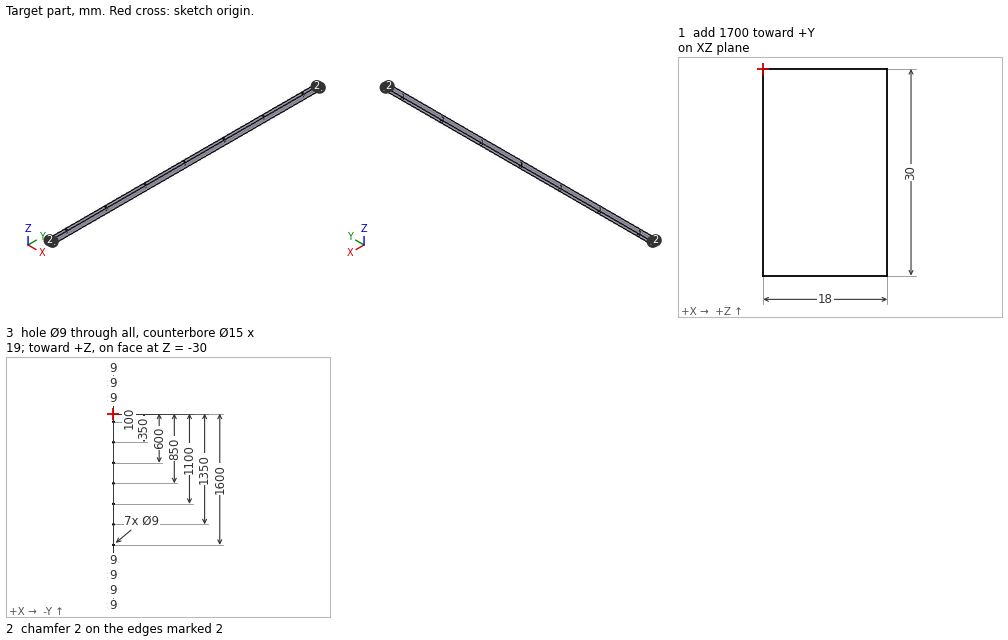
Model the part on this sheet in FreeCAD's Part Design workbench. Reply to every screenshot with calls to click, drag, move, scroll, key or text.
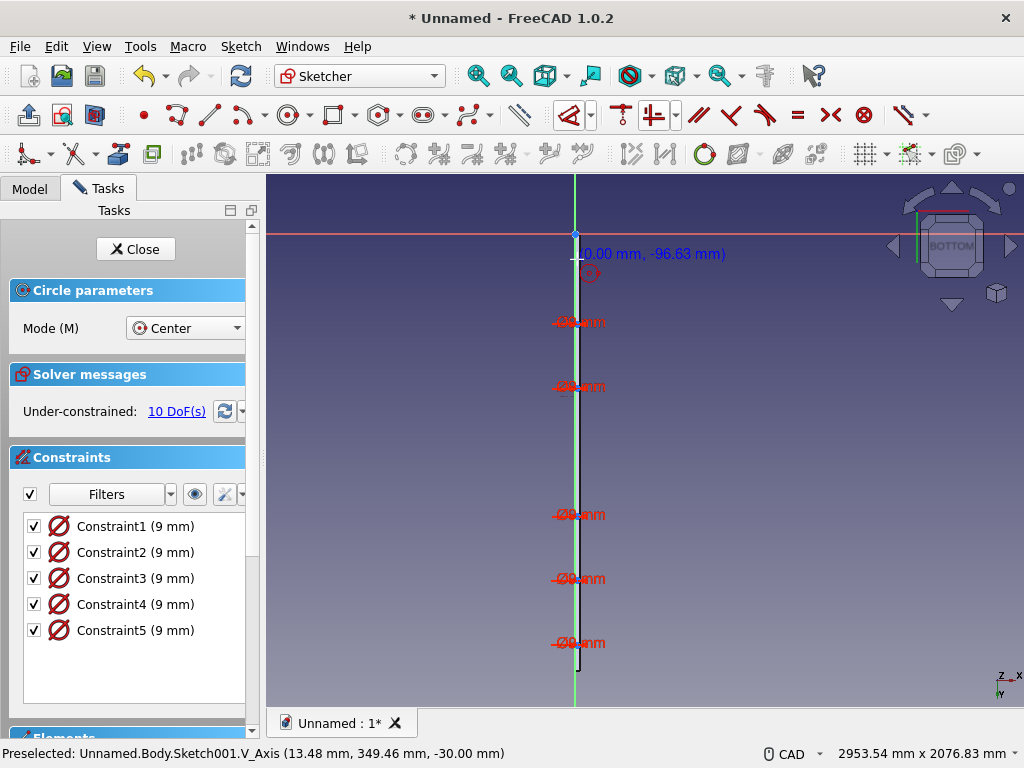
scroll(577, 260, up, 10)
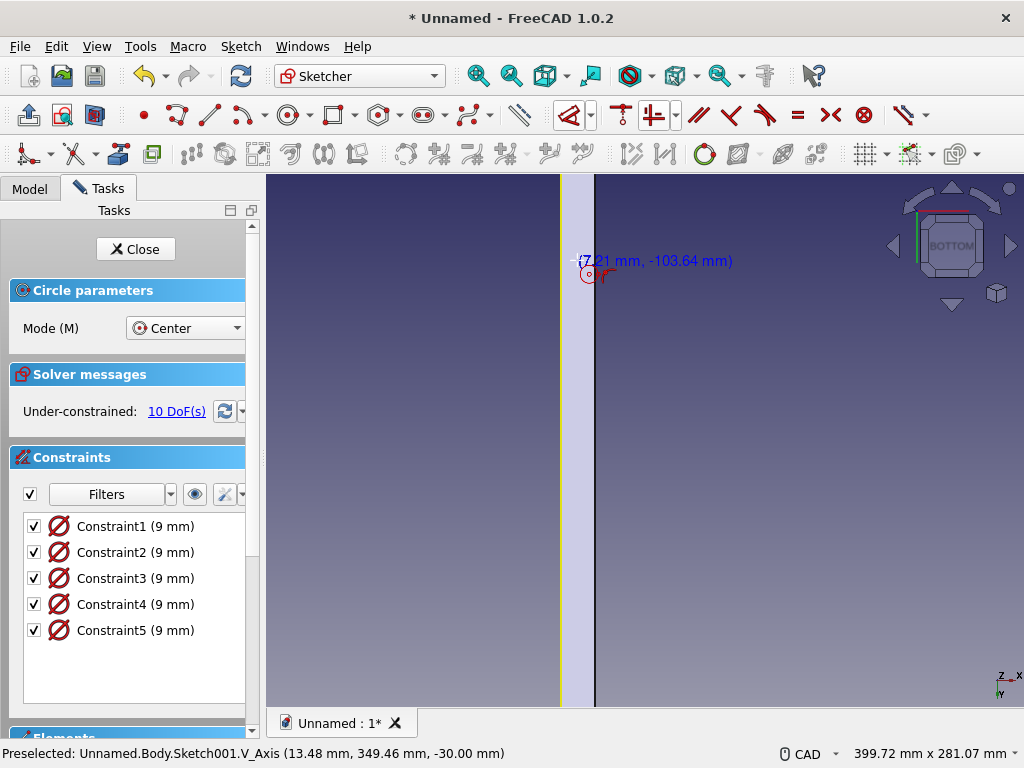
click(578, 259)
move(584, 253)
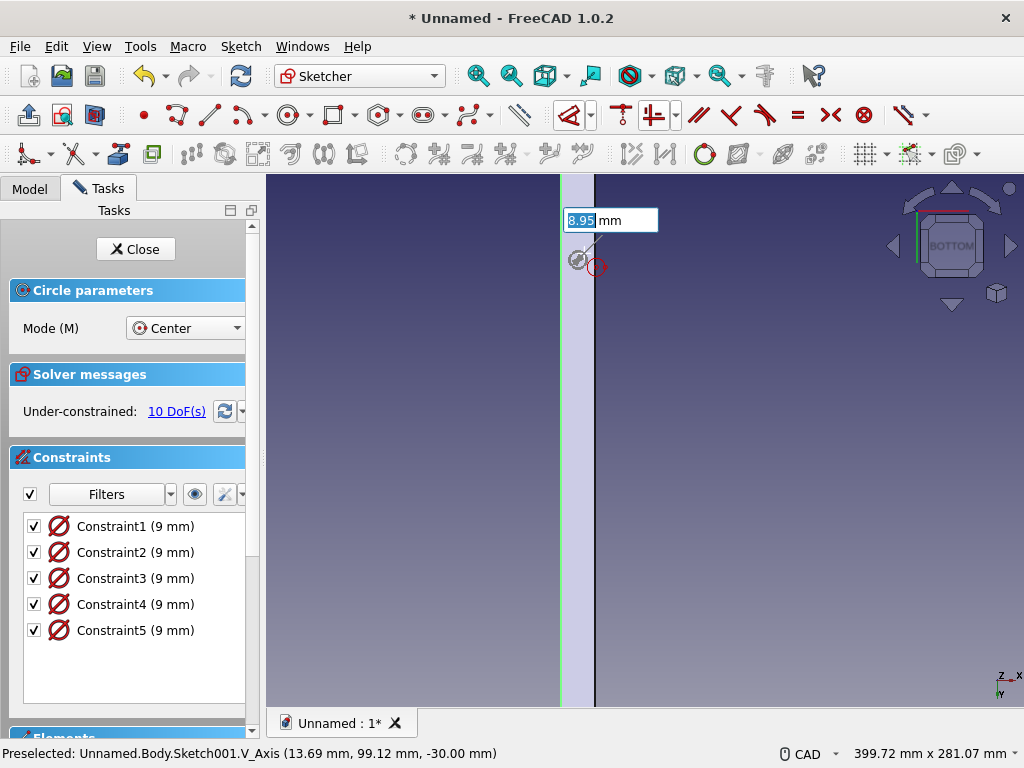
text(9)
key(Return)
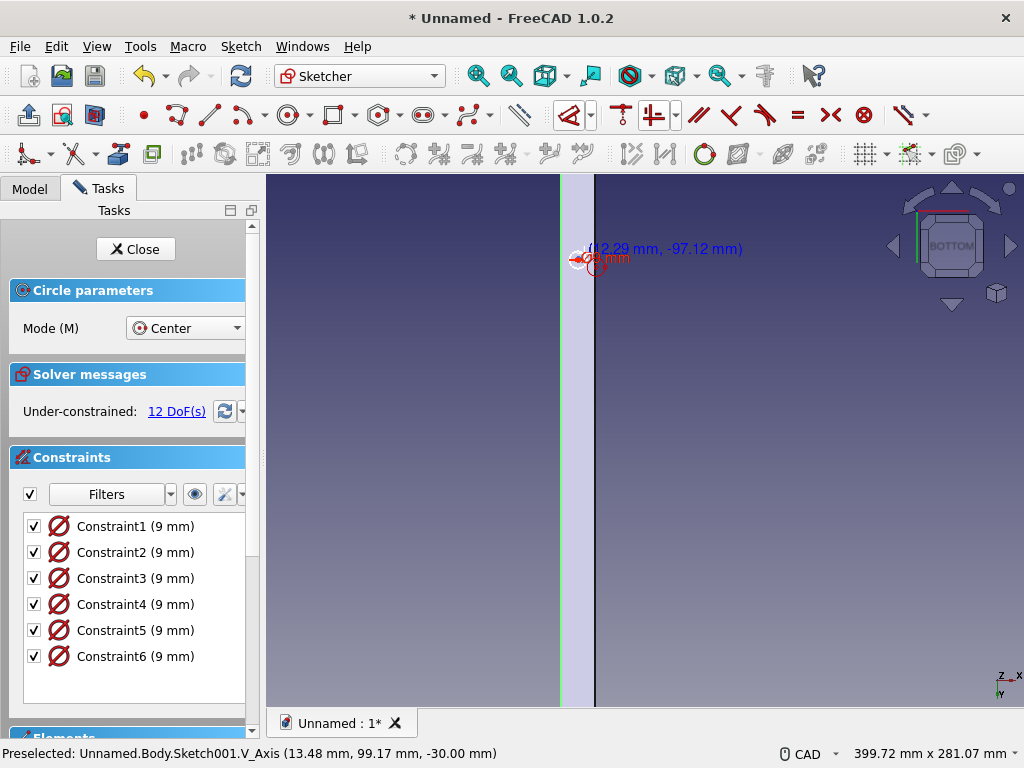
scroll(577, 297, down, 11)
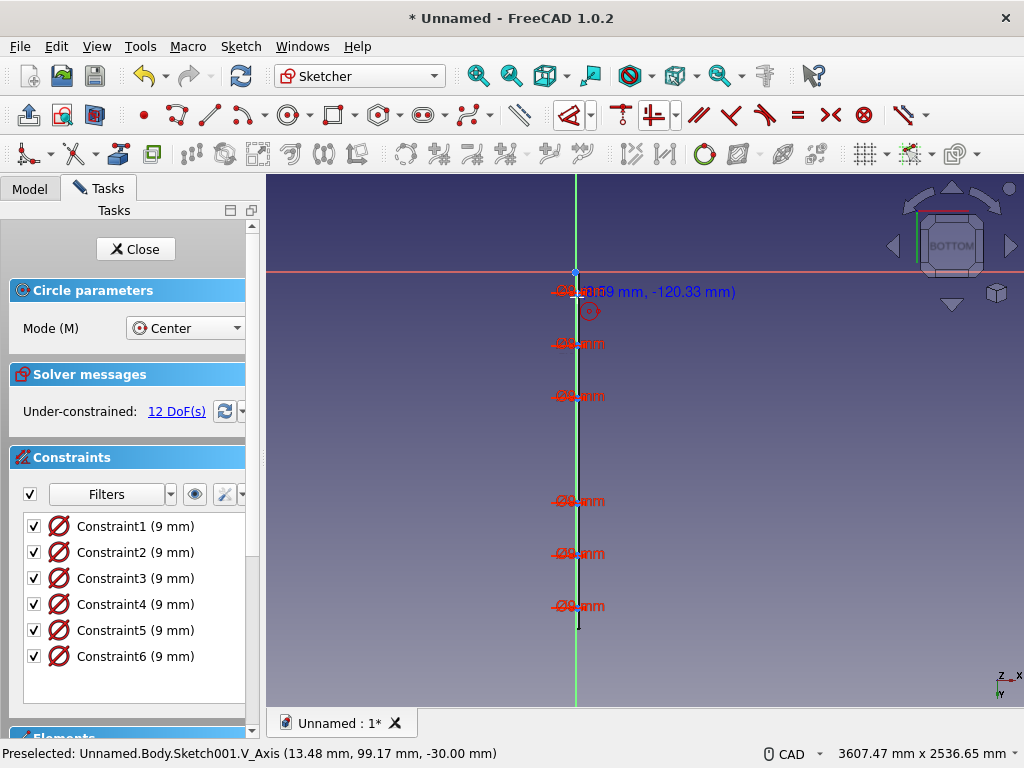
scroll(577, 451, up, 16)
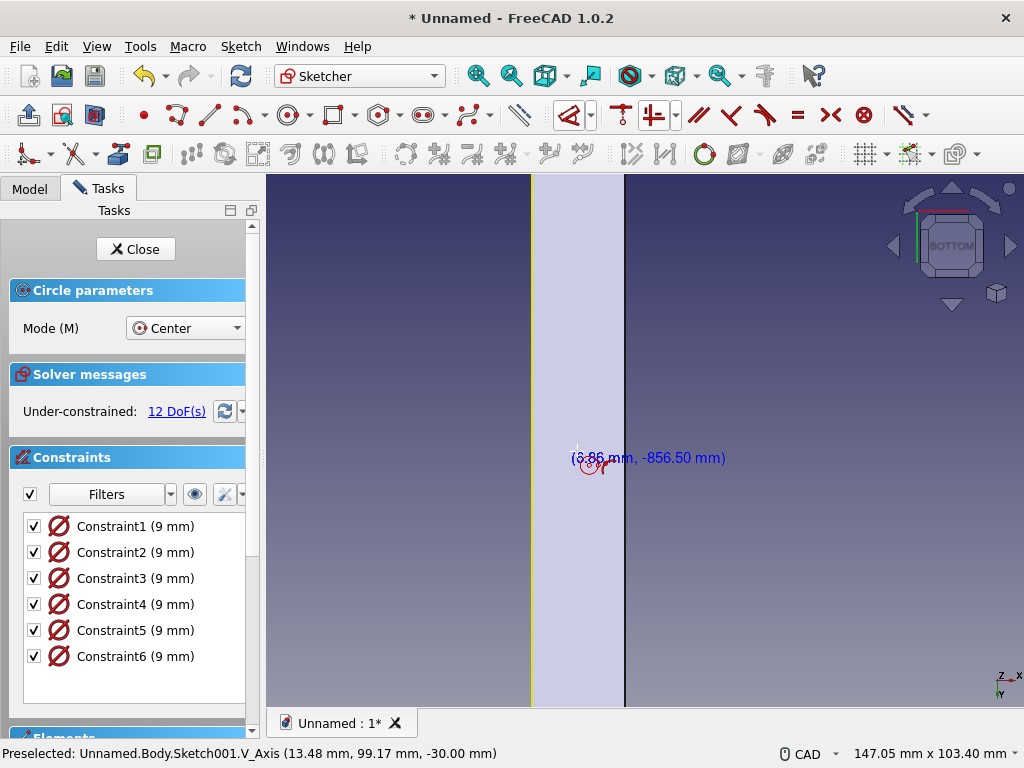
scroll(577, 454, down, 15)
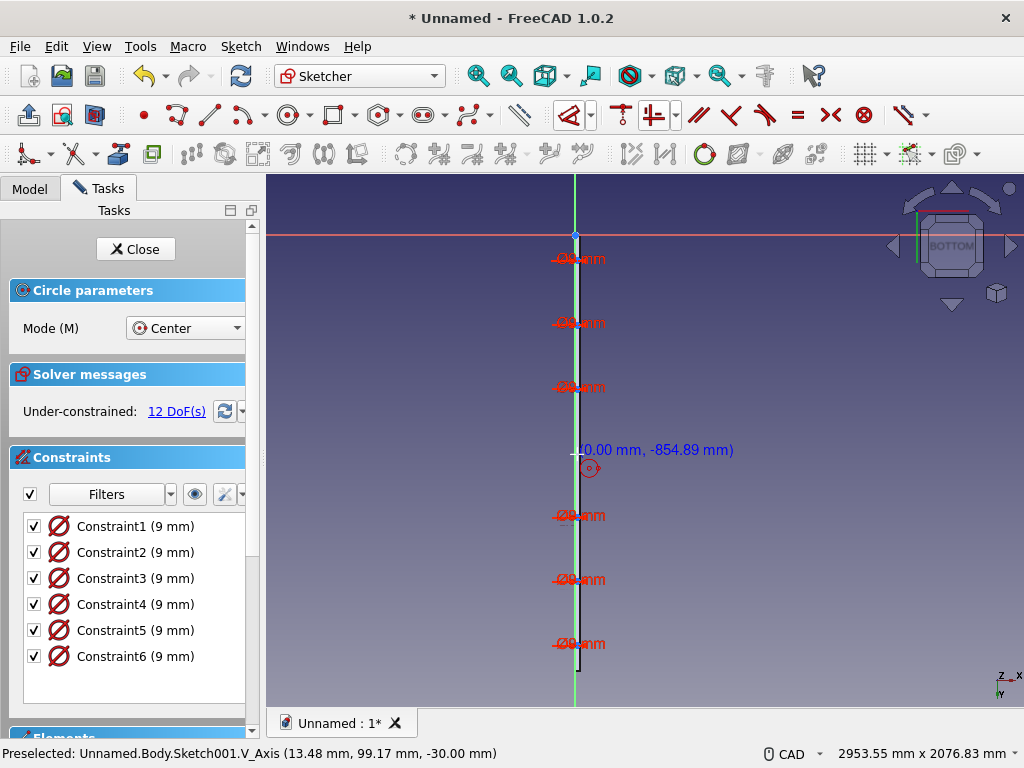
scroll(577, 453, up, 10)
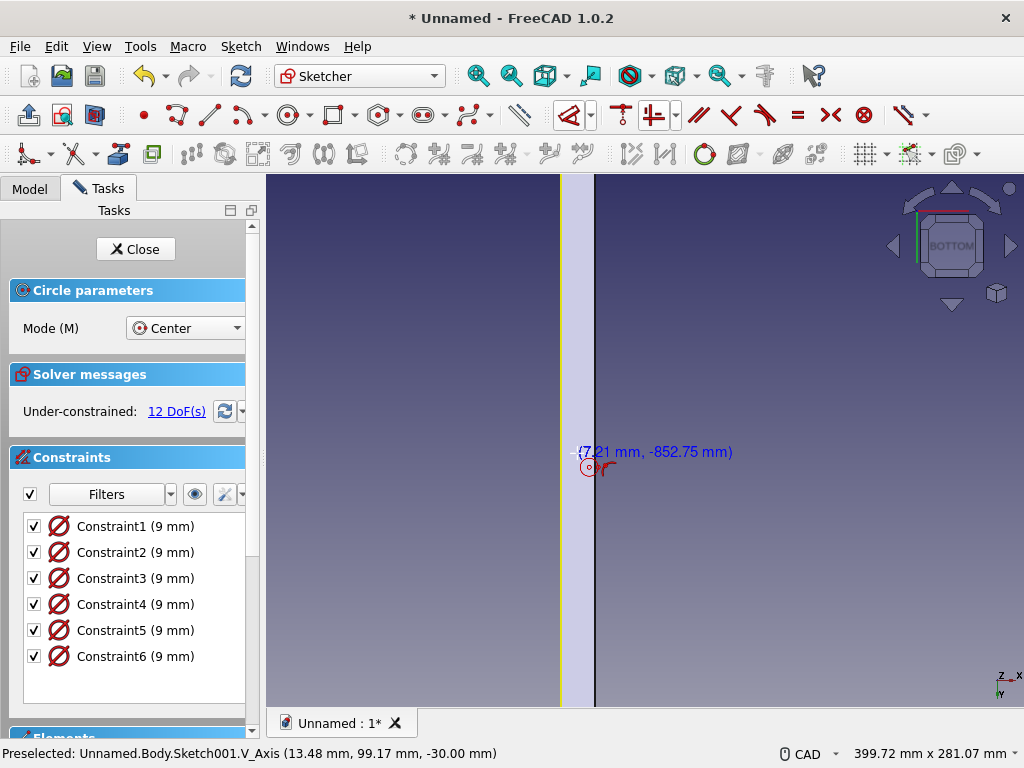
click(578, 452)
move(584, 446)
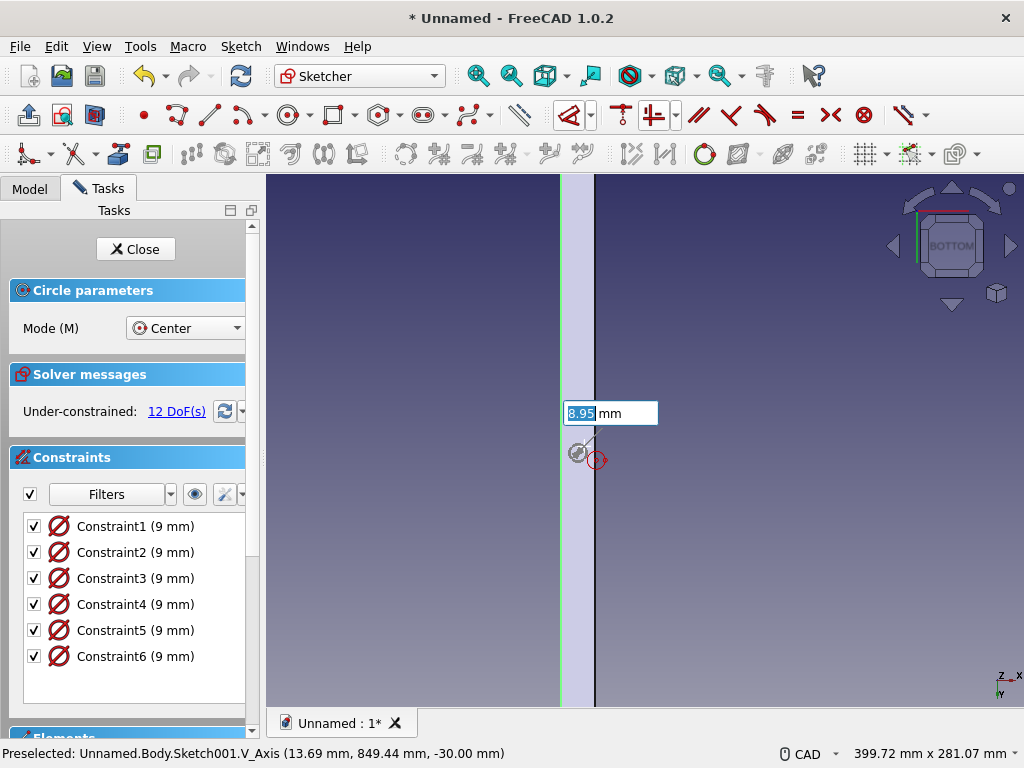
text(9)
key(Return)
key(Escape)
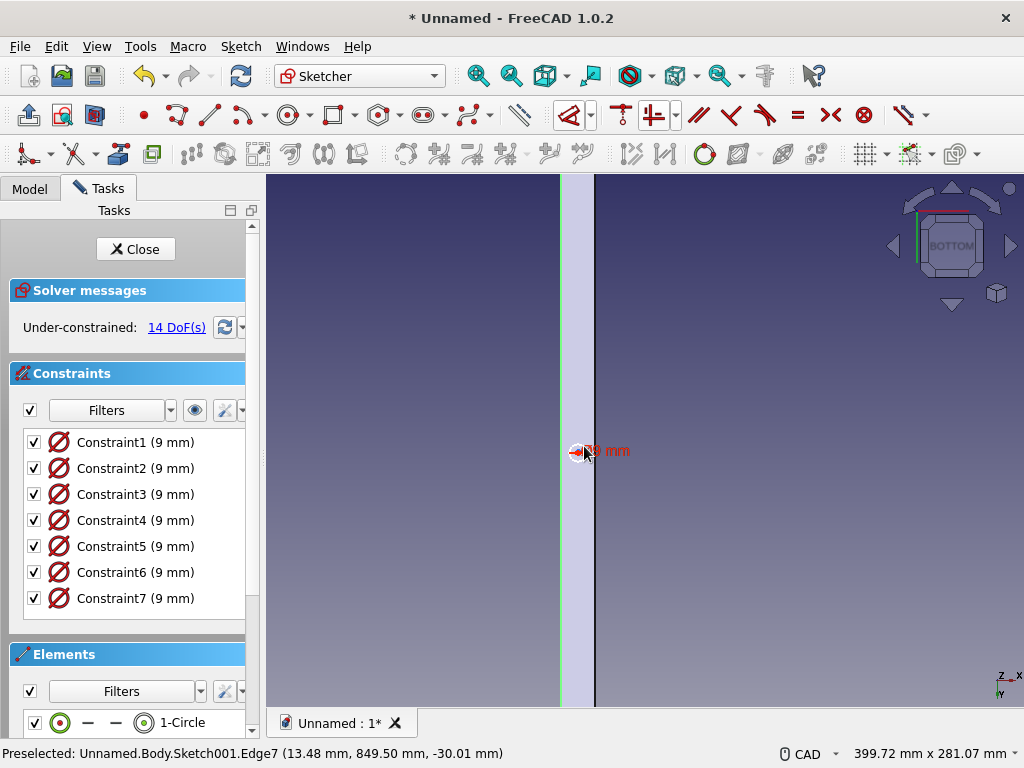
click(568, 116)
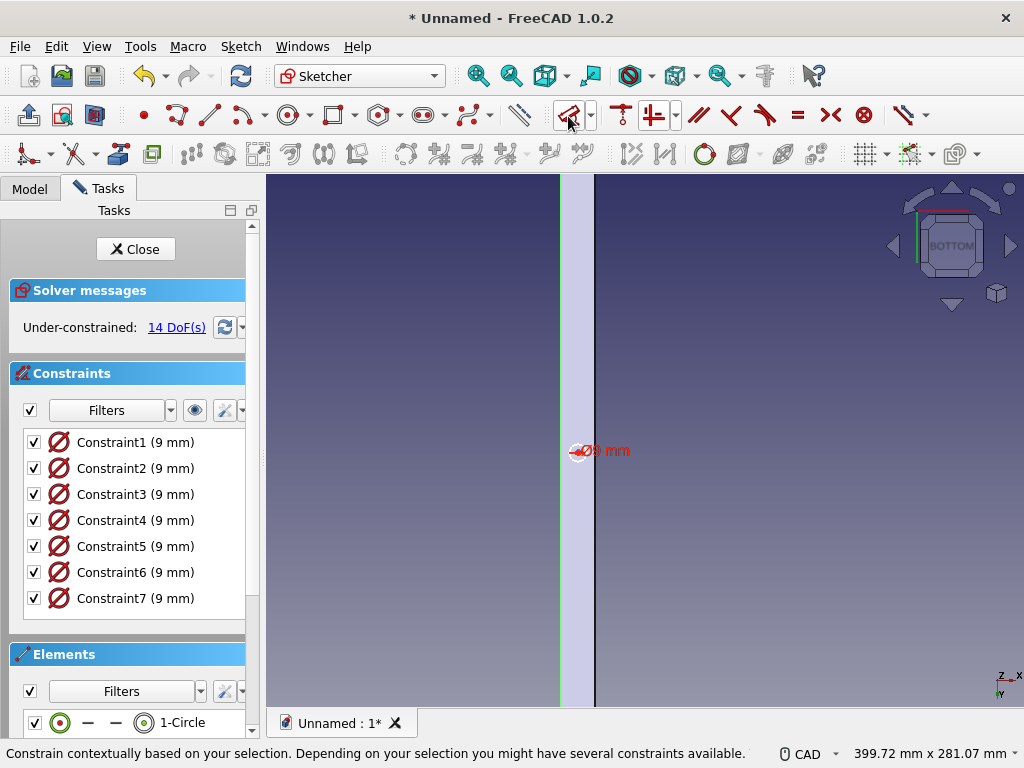
scroll(577, 450, down, 11)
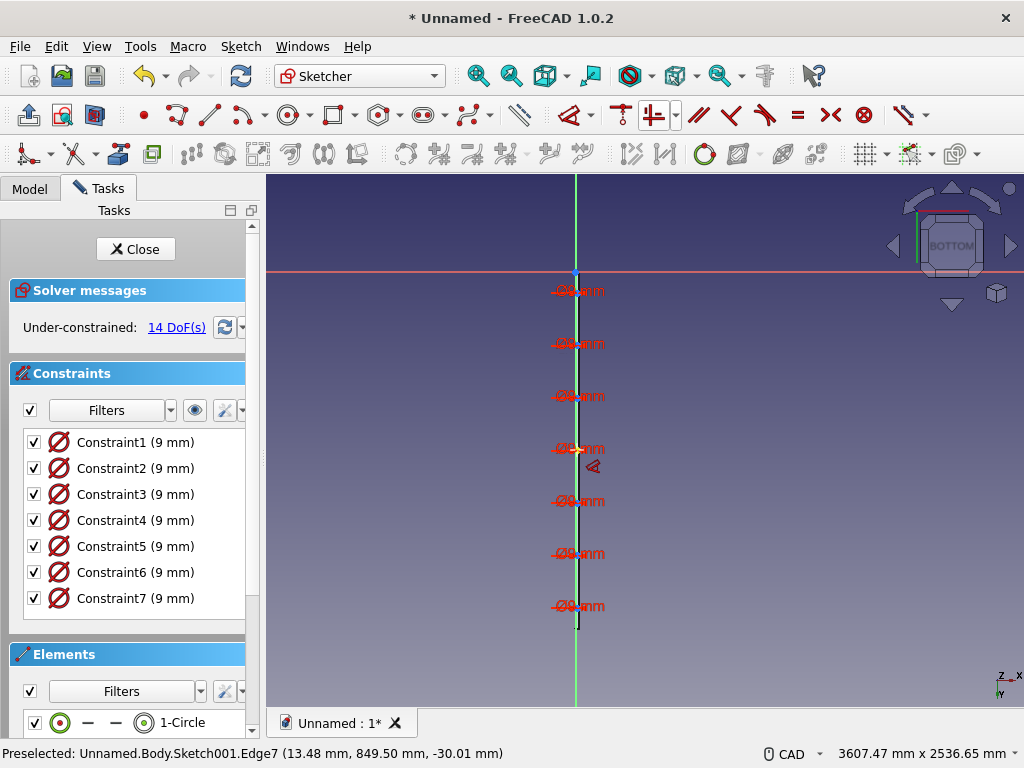
scroll(577, 608, up, 16)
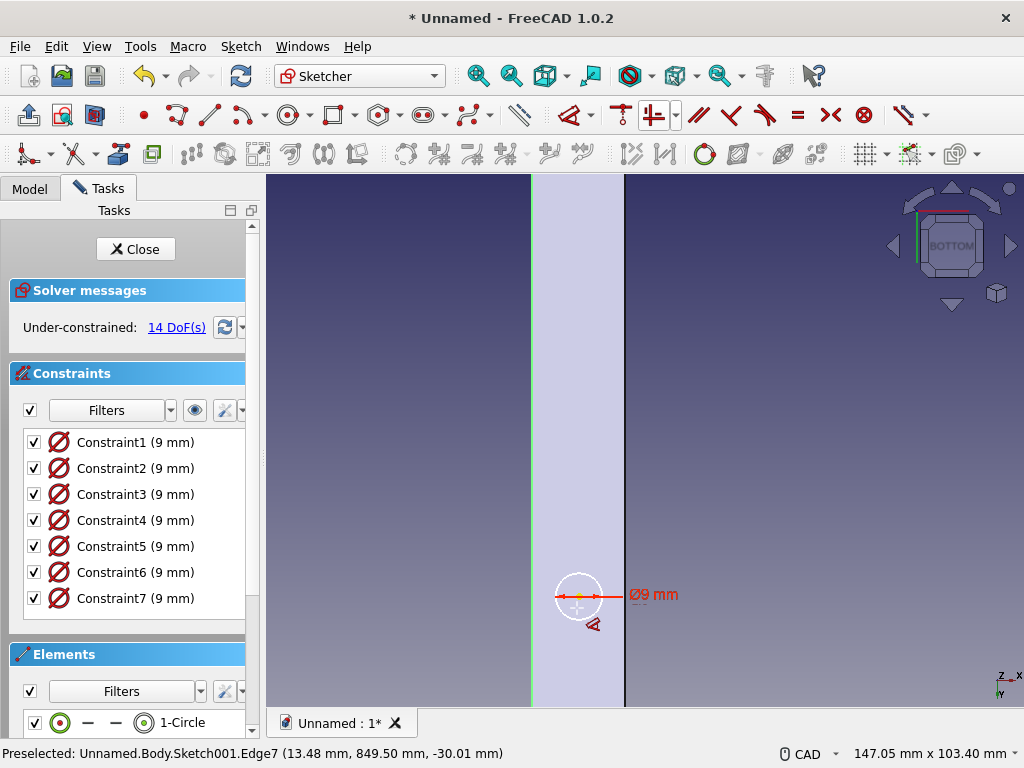
click(579, 597)
click(556, 631)